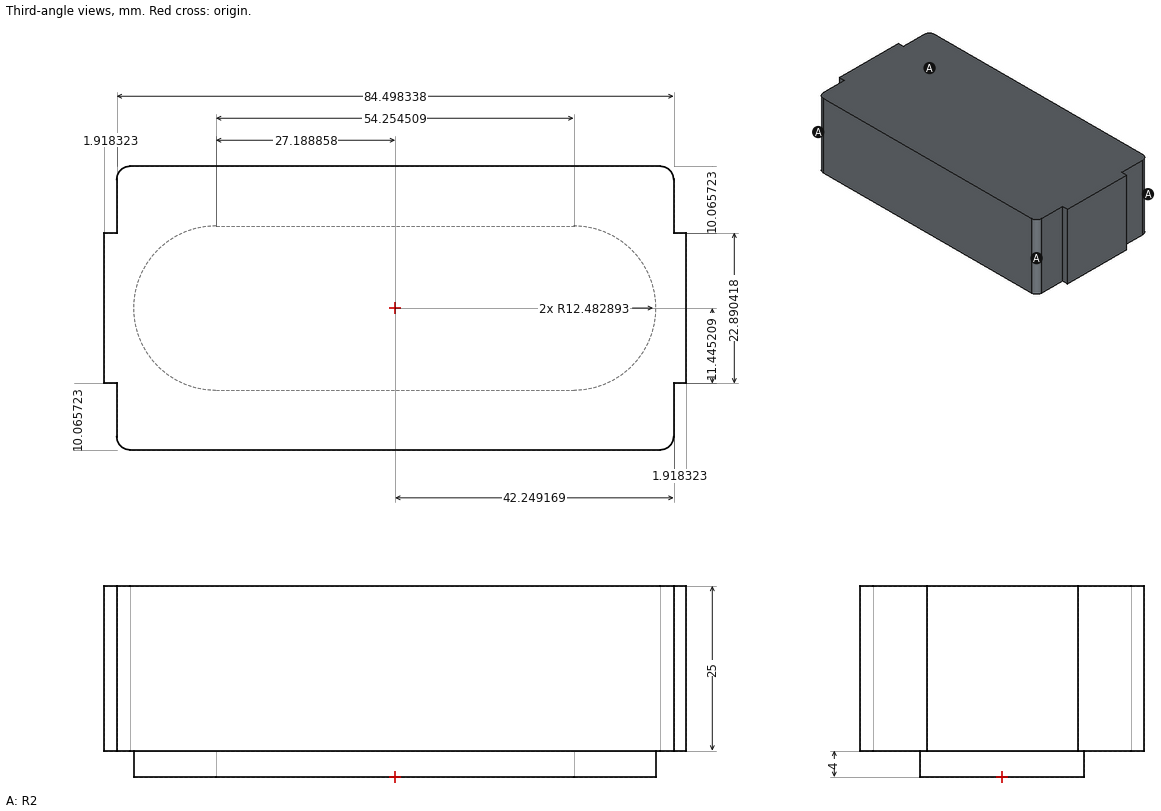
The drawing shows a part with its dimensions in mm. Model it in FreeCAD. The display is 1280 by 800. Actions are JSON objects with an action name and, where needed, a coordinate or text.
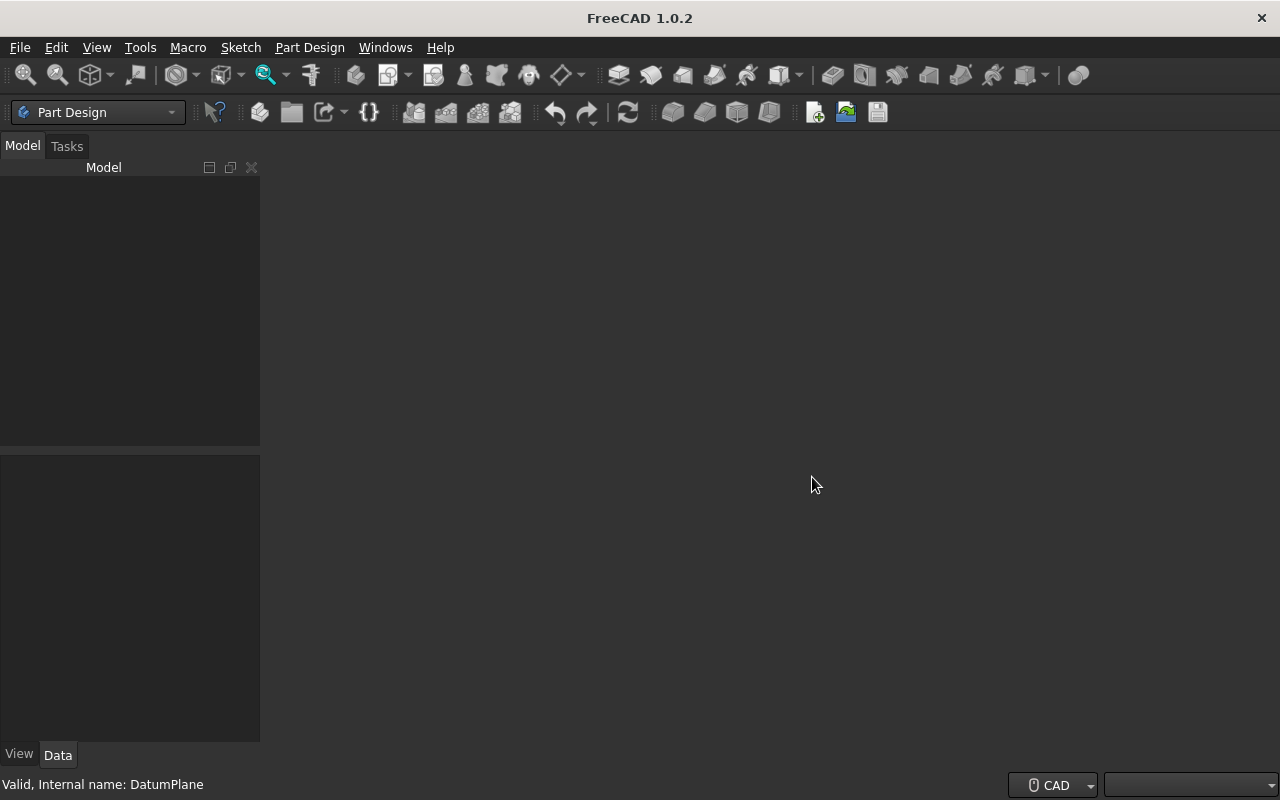
{"action": "left_click", "coordinate": [814, 112]}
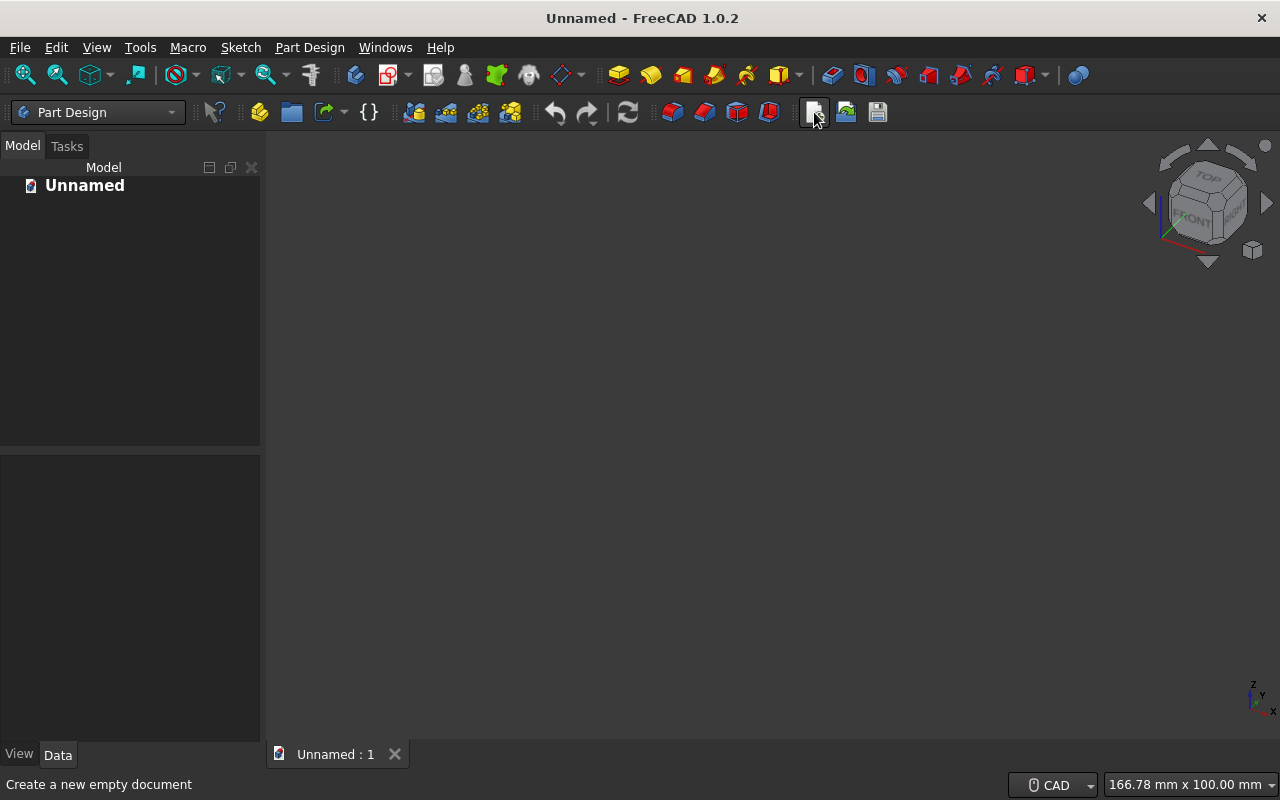
{"action": "left_click", "coordinate": [388, 76]}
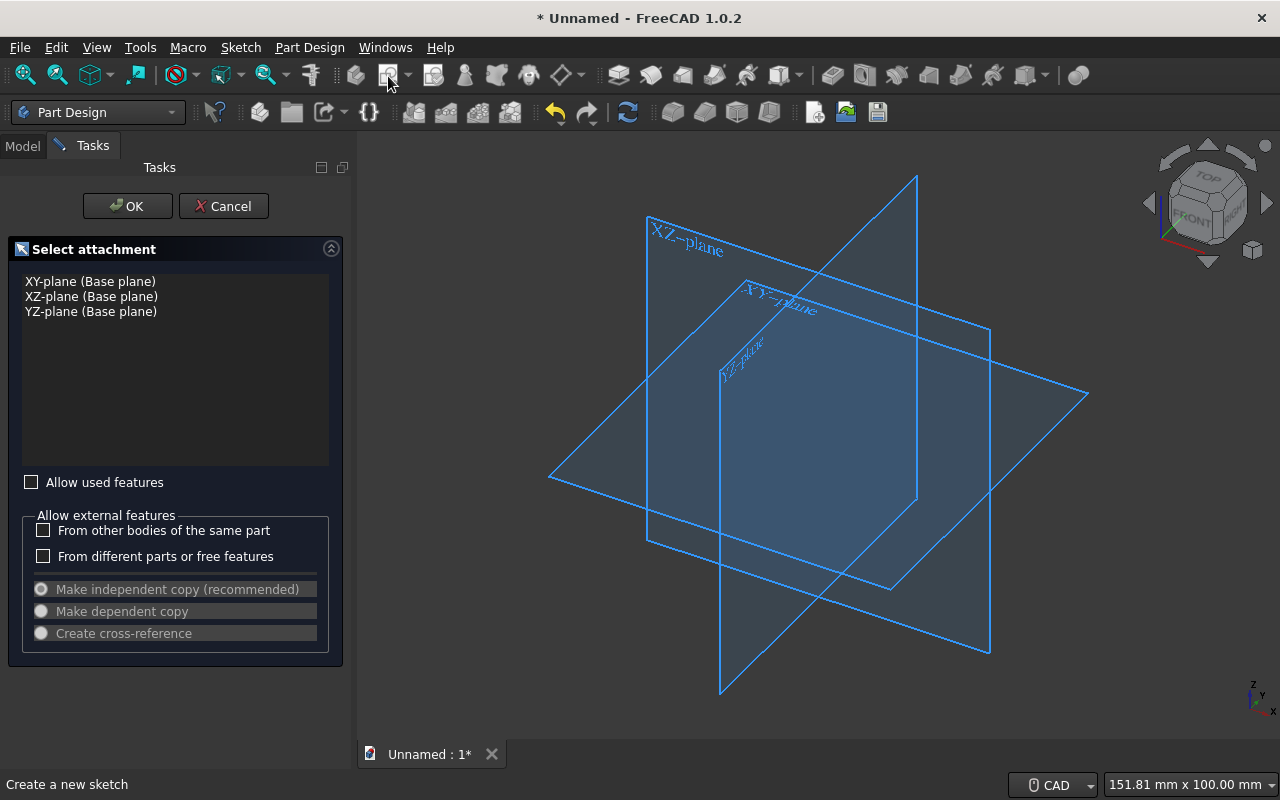
{"action": "left_click", "coordinate": [82, 282]}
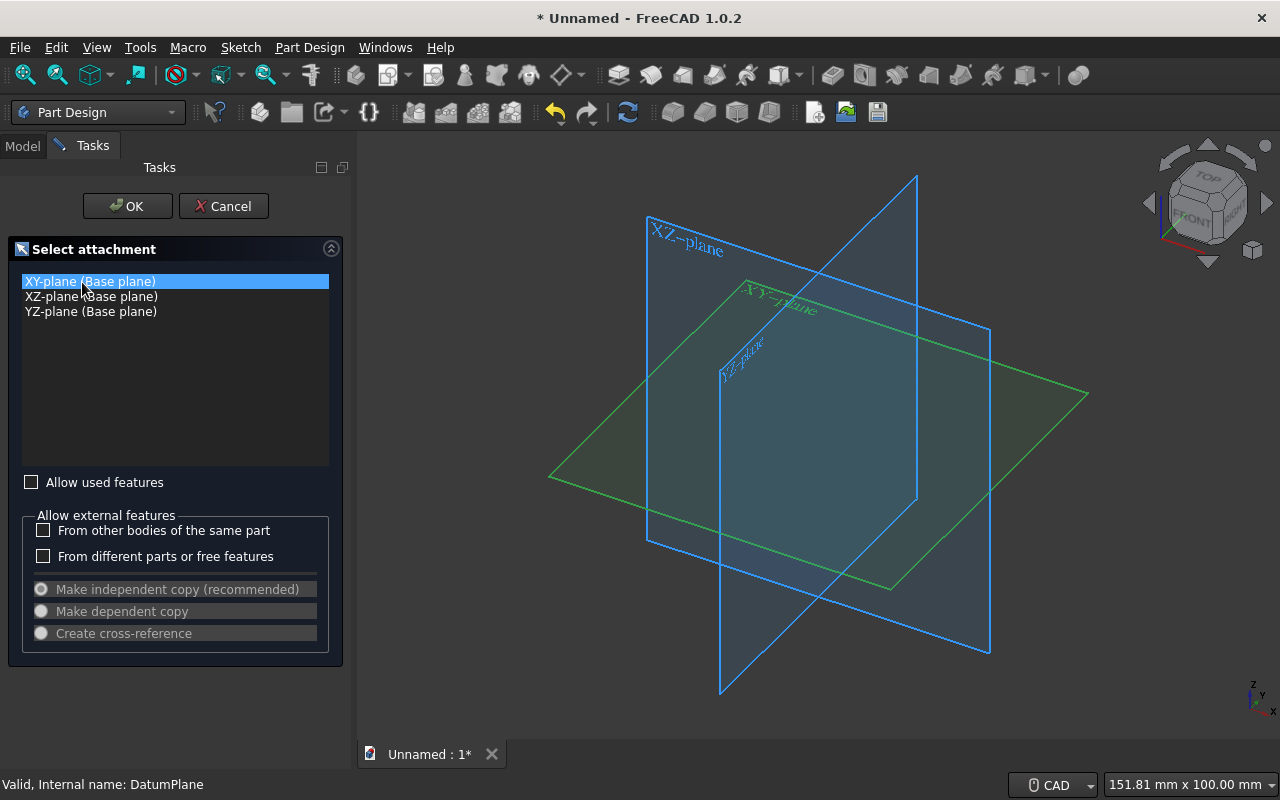
{"action": "left_click", "coordinate": [128, 206]}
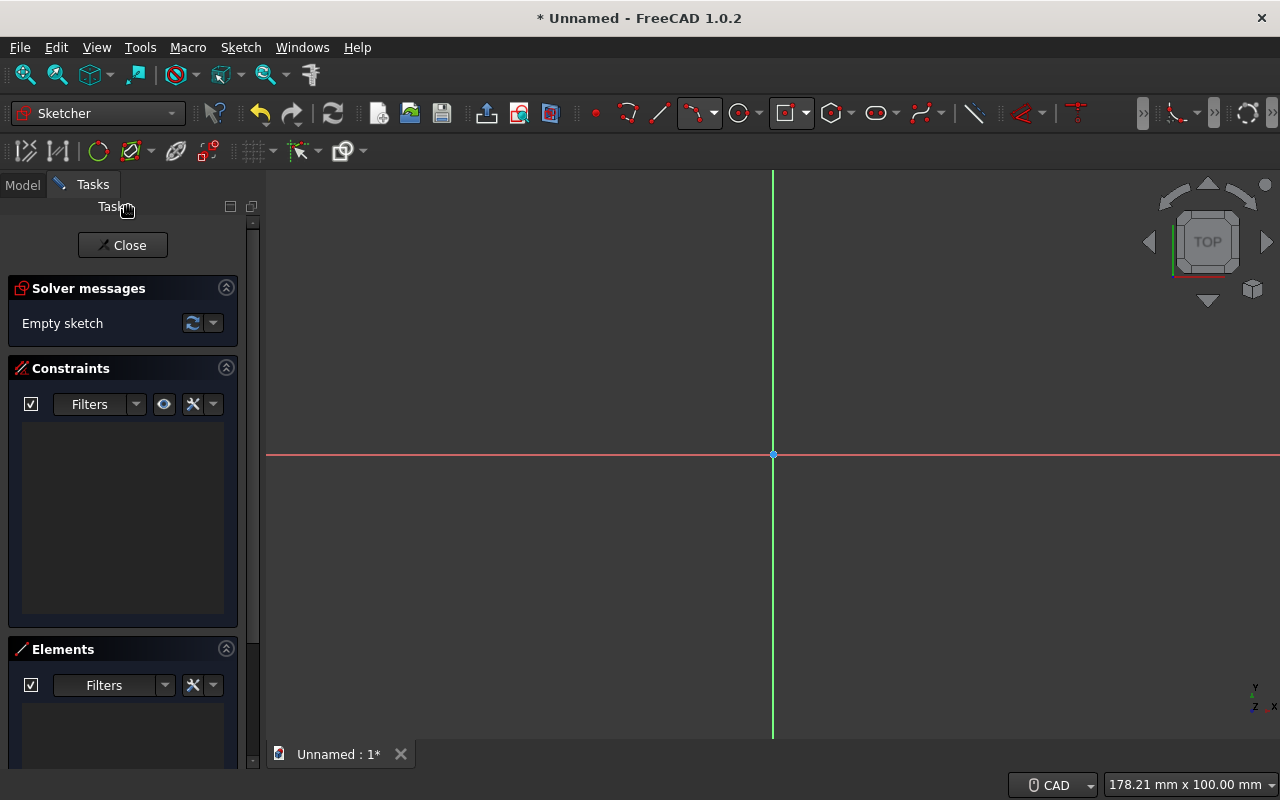
{"action": "left_click", "coordinate": [876, 114]}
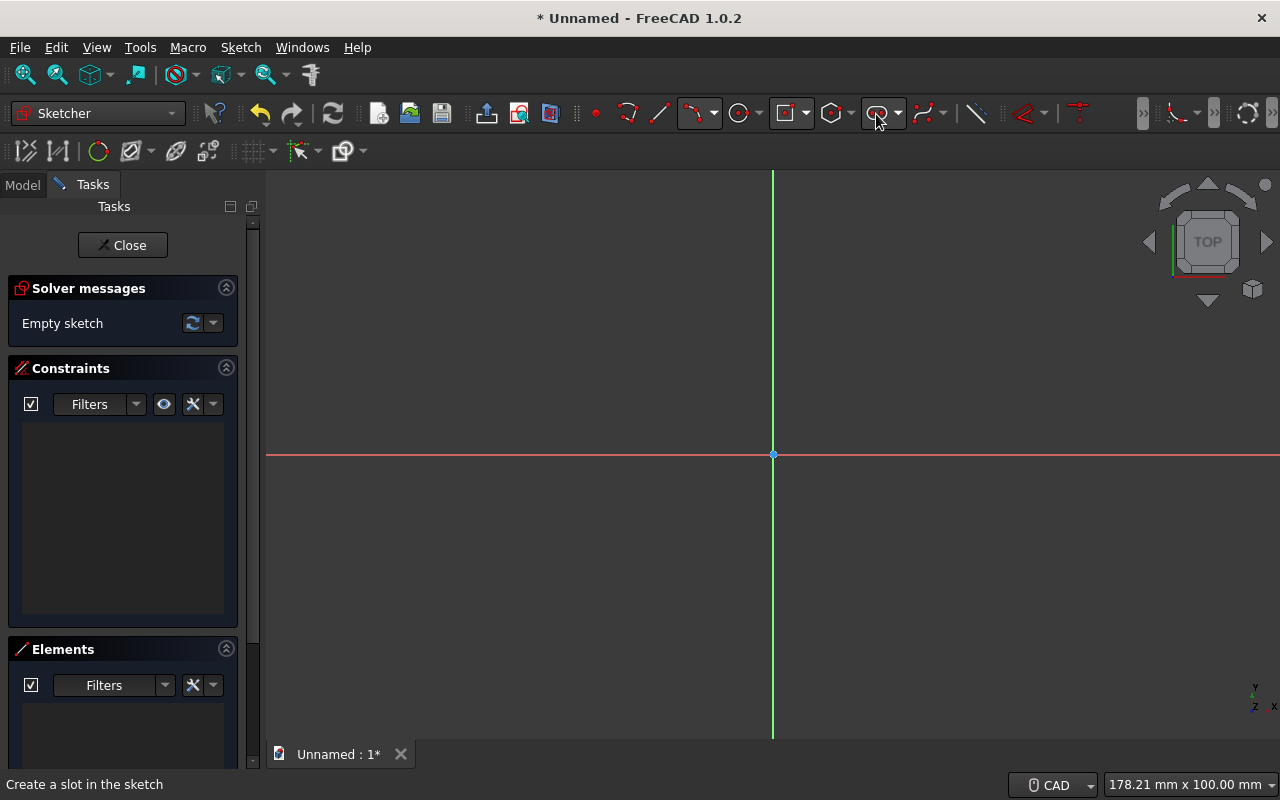
{"action": "left_click", "coordinate": [618, 454]}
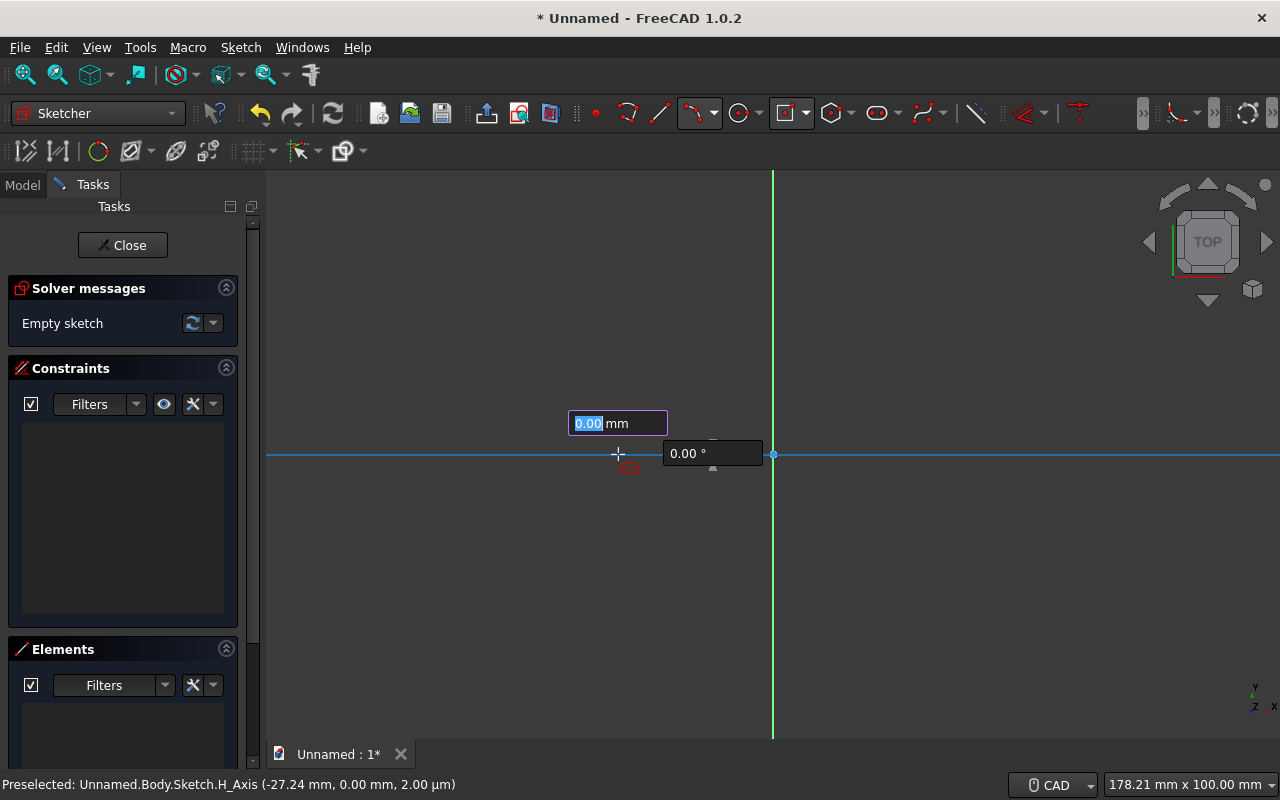
{"action": "left_click", "coordinate": [927, 446]}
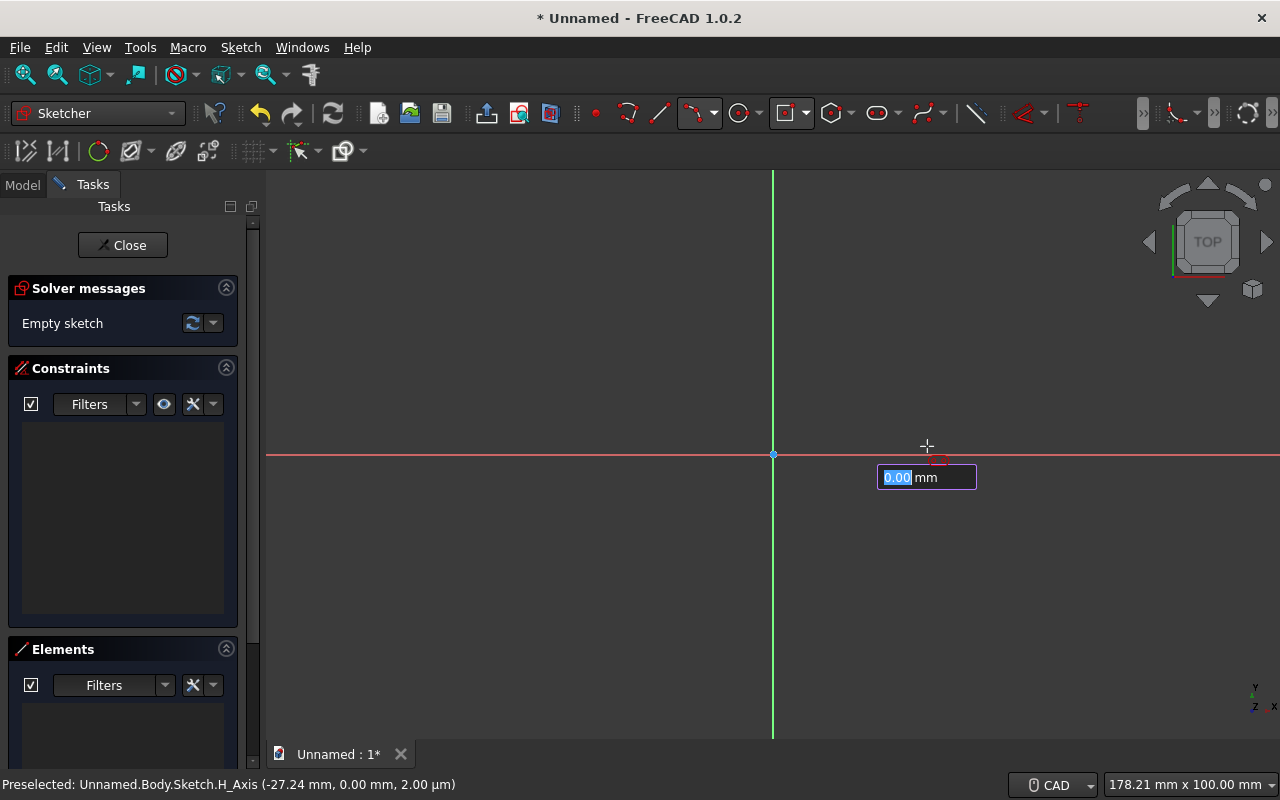
{"action": "left_click", "coordinate": [726, 526]}
{"action": "key", "text": "Escape"}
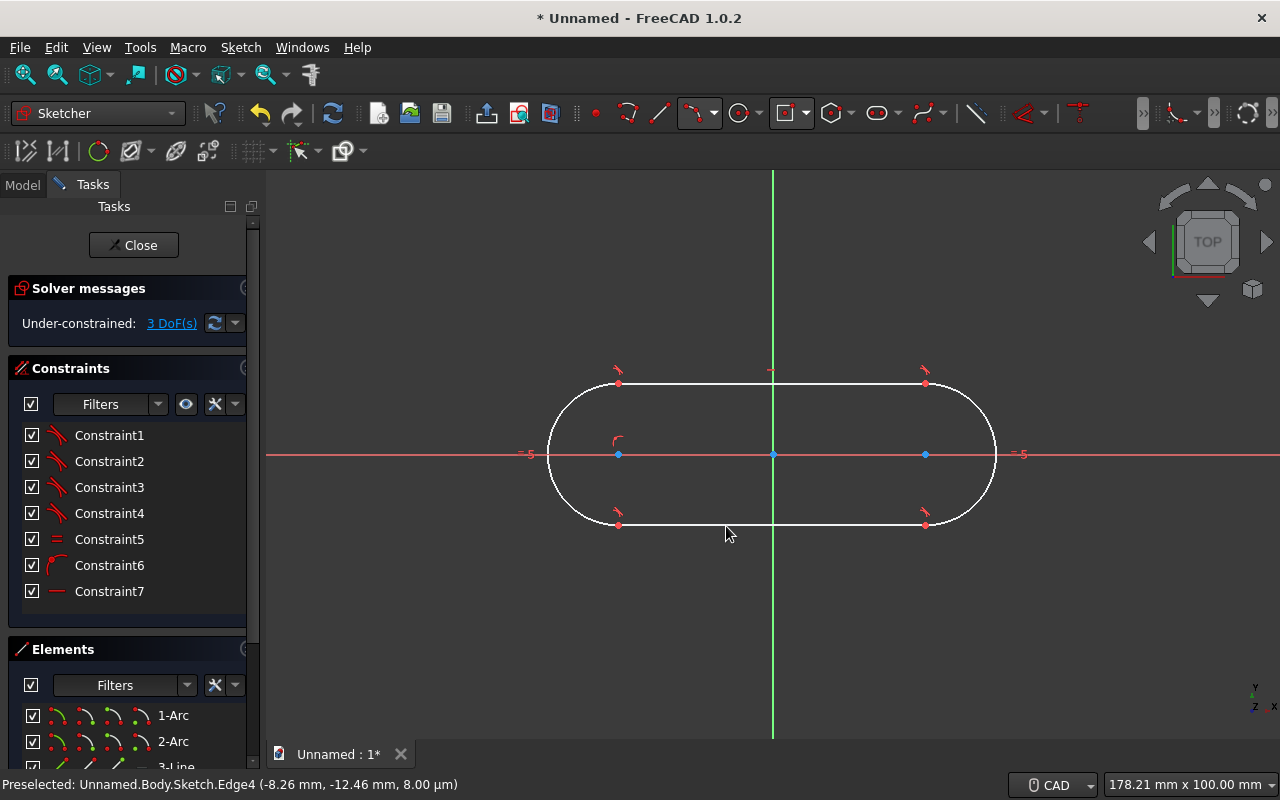
{"action": "left_click", "coordinate": [1024, 114]}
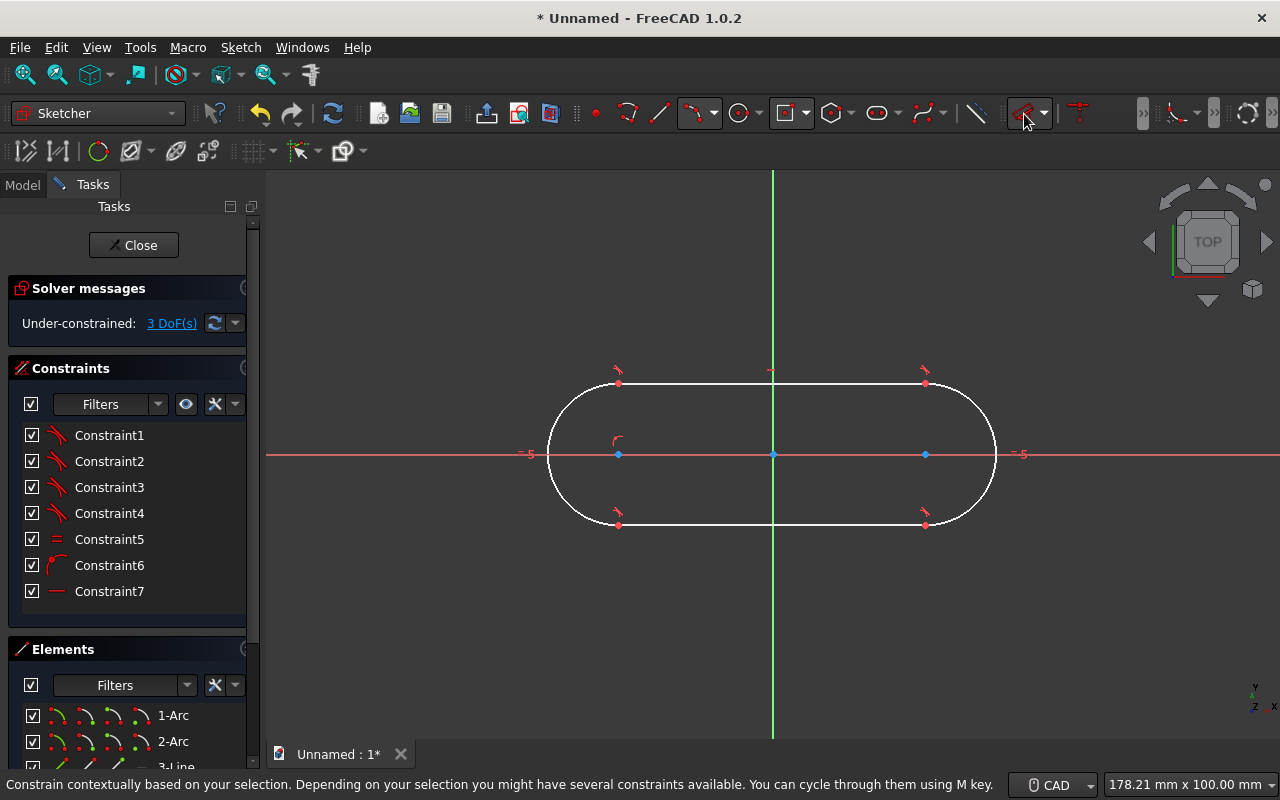
{"action": "left_click", "coordinate": [561, 413]}
{"action": "left_click", "coordinate": [535, 394]}